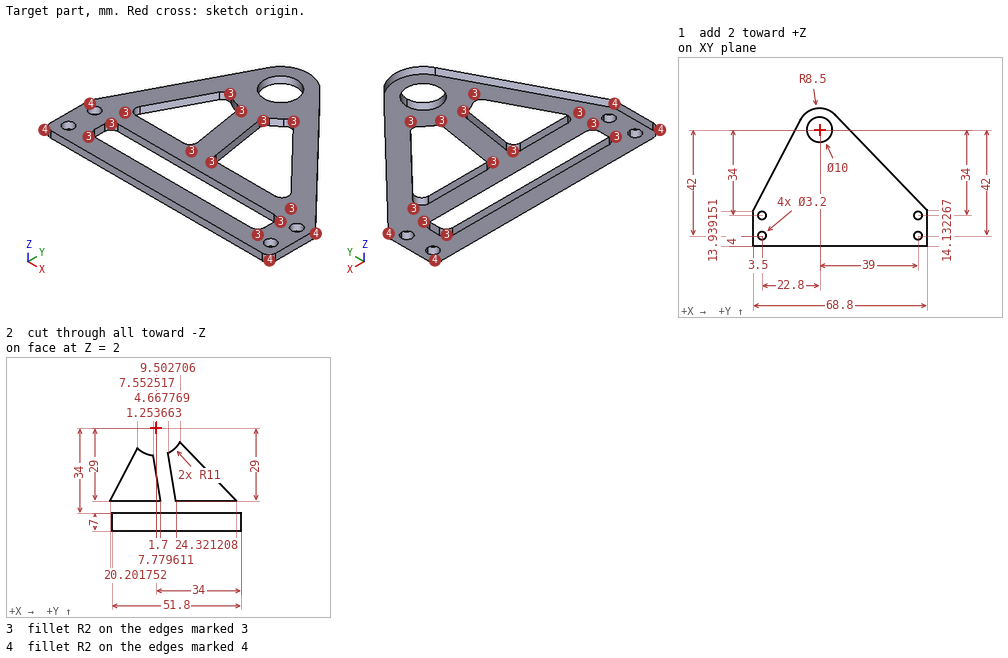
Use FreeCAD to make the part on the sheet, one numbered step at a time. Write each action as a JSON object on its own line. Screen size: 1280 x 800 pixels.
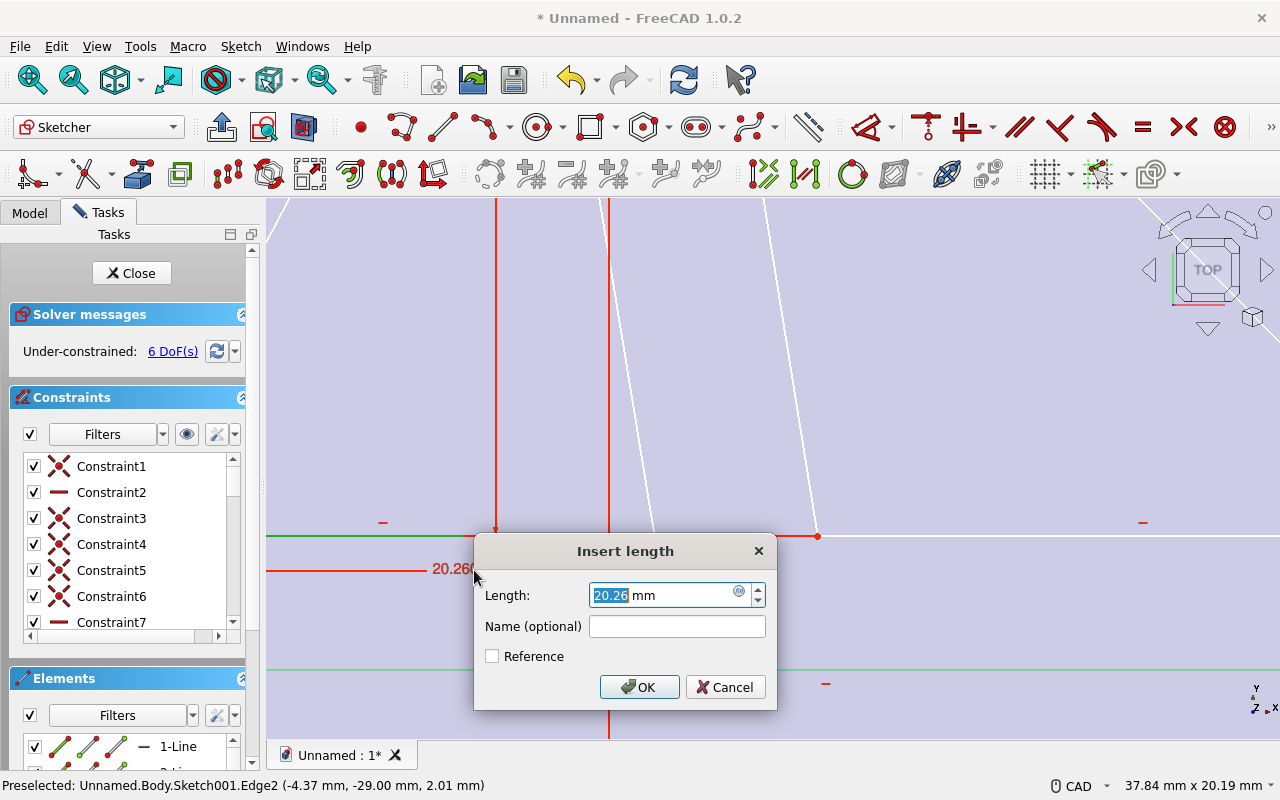
{"action": "type", "text": "20.201752"}
{"action": "key", "text": "Return"}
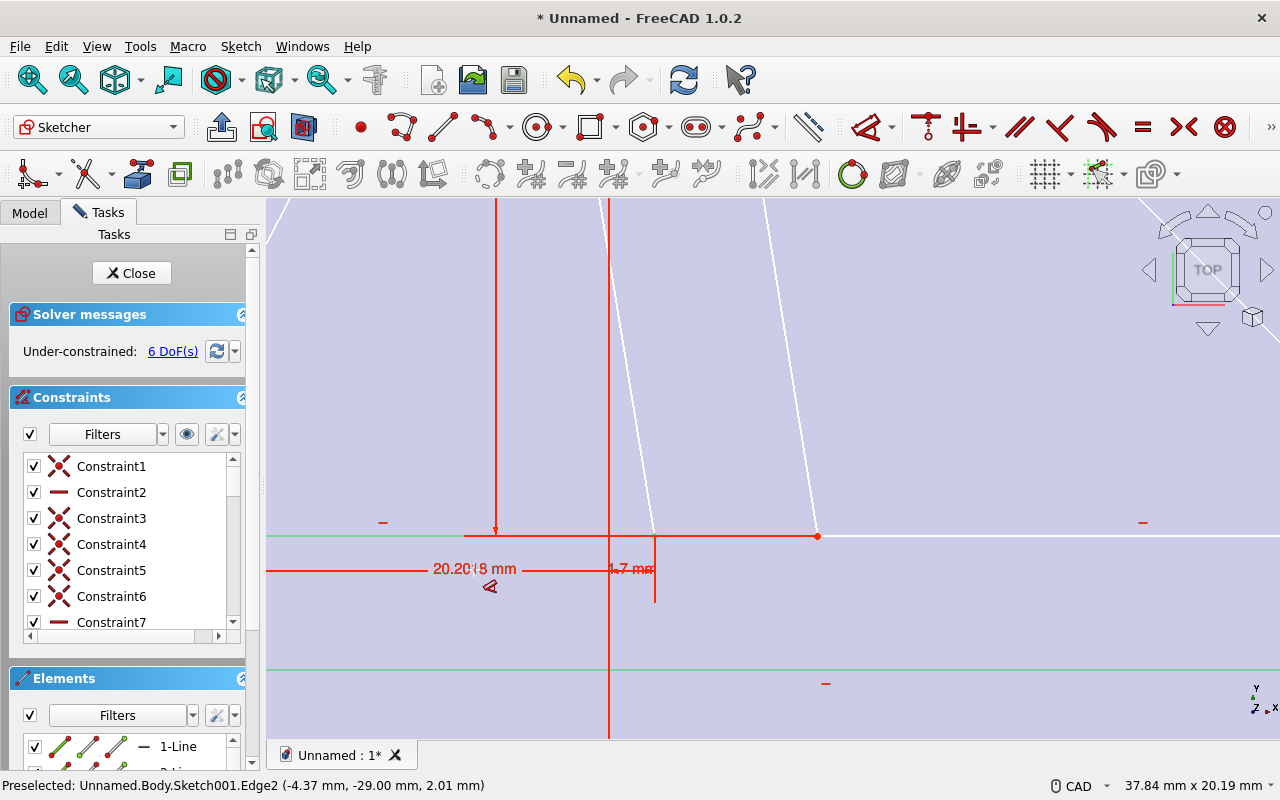
{"action": "left_click", "coordinate": [1013, 536]}
{"action": "left_click", "coordinate": [966, 570]}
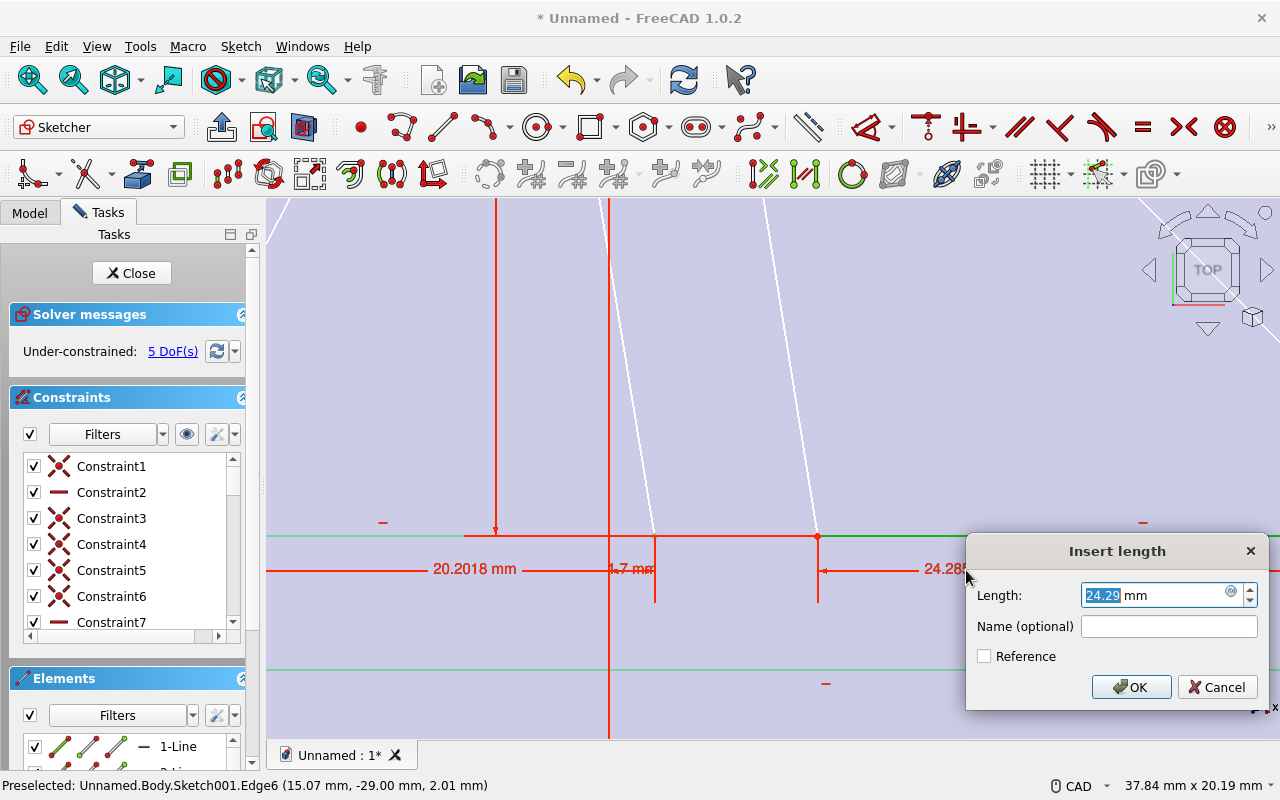
{"action": "type", "text": "24.321208"}
{"action": "key", "text": "Return"}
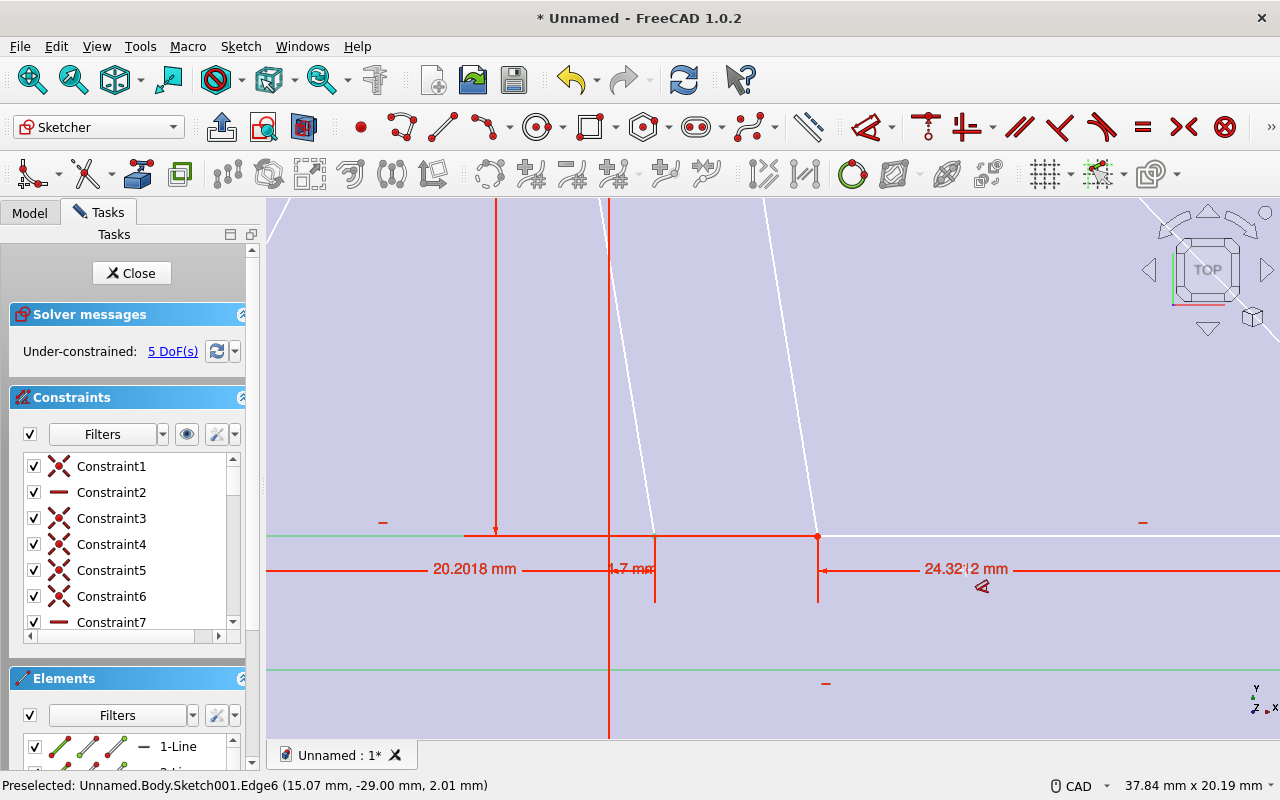
{"action": "scroll", "coordinate": [656, 537], "scroll_direction": "down", "scroll_amount": 6}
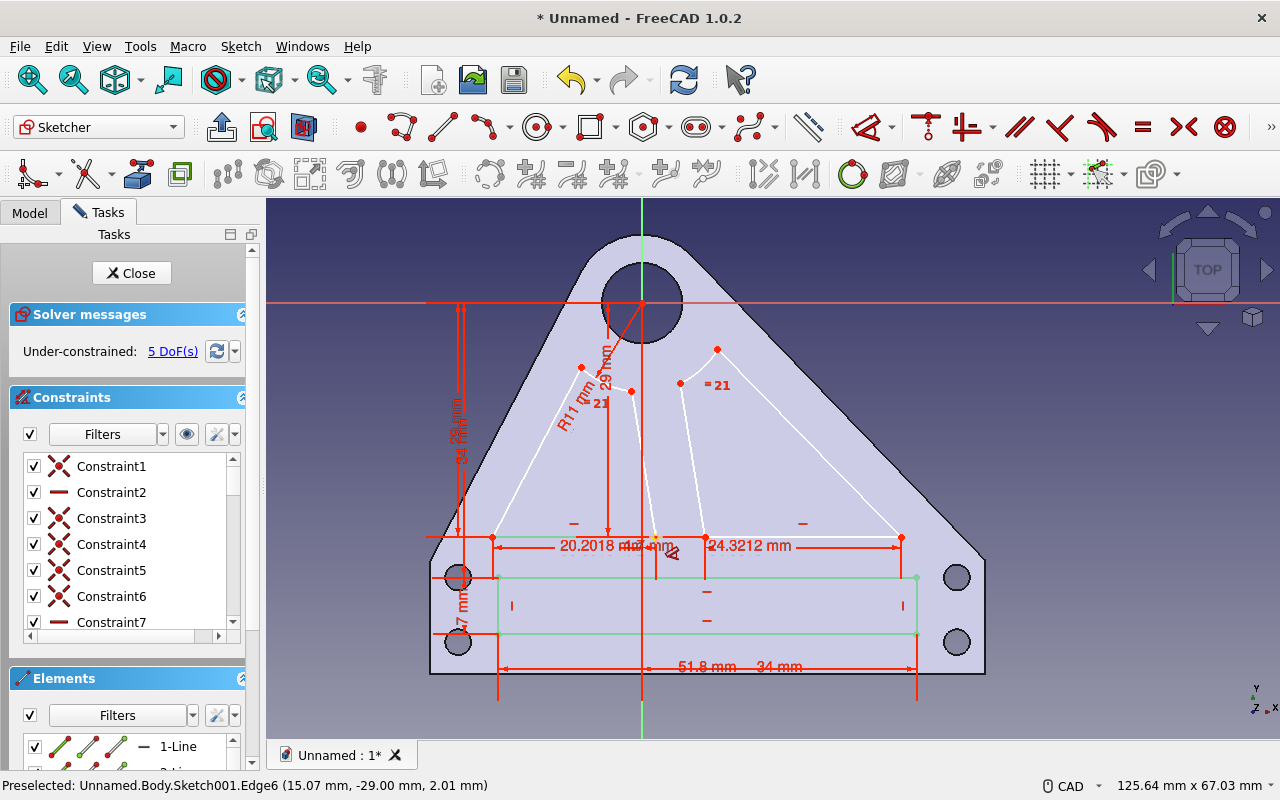
{"action": "left_click", "coordinate": [581, 368]}
{"action": "left_click", "coordinate": [612, 269]}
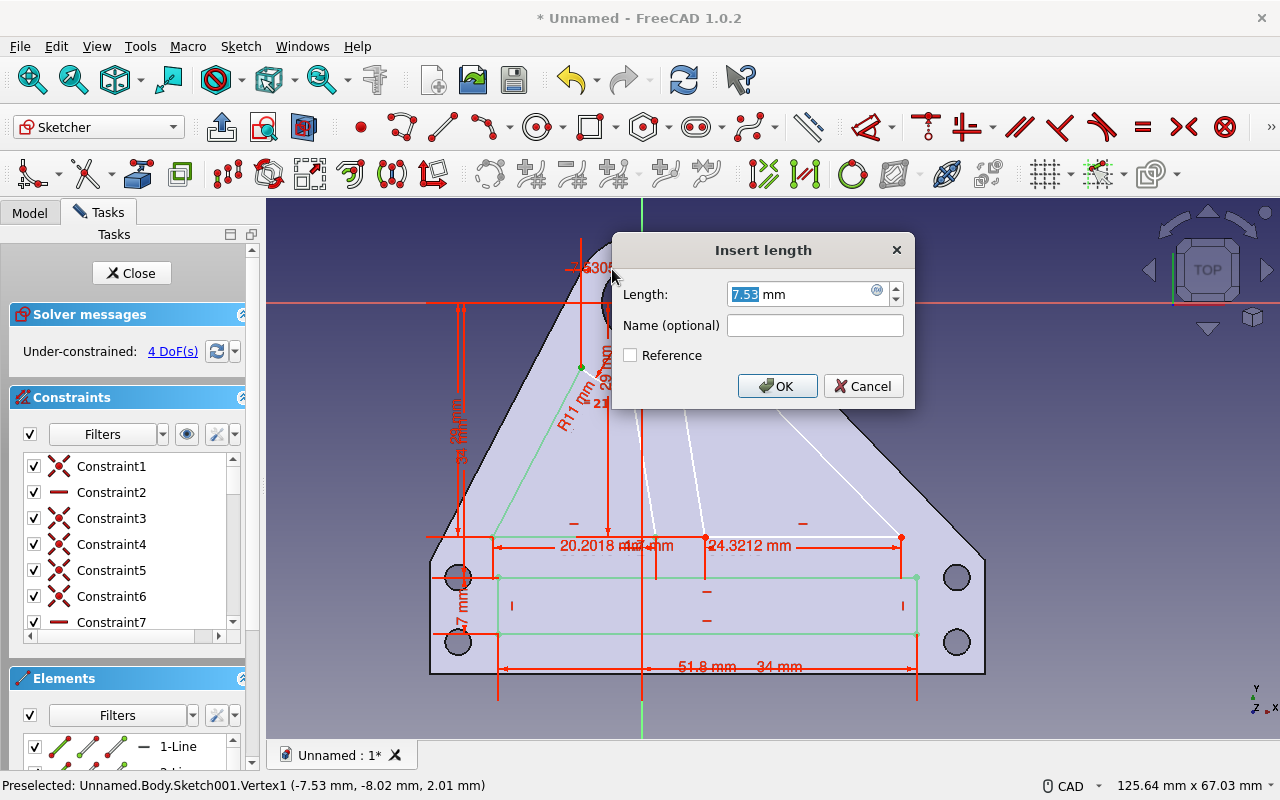
{"action": "type", "text": "7.552517"}
{"action": "key", "text": "Return"}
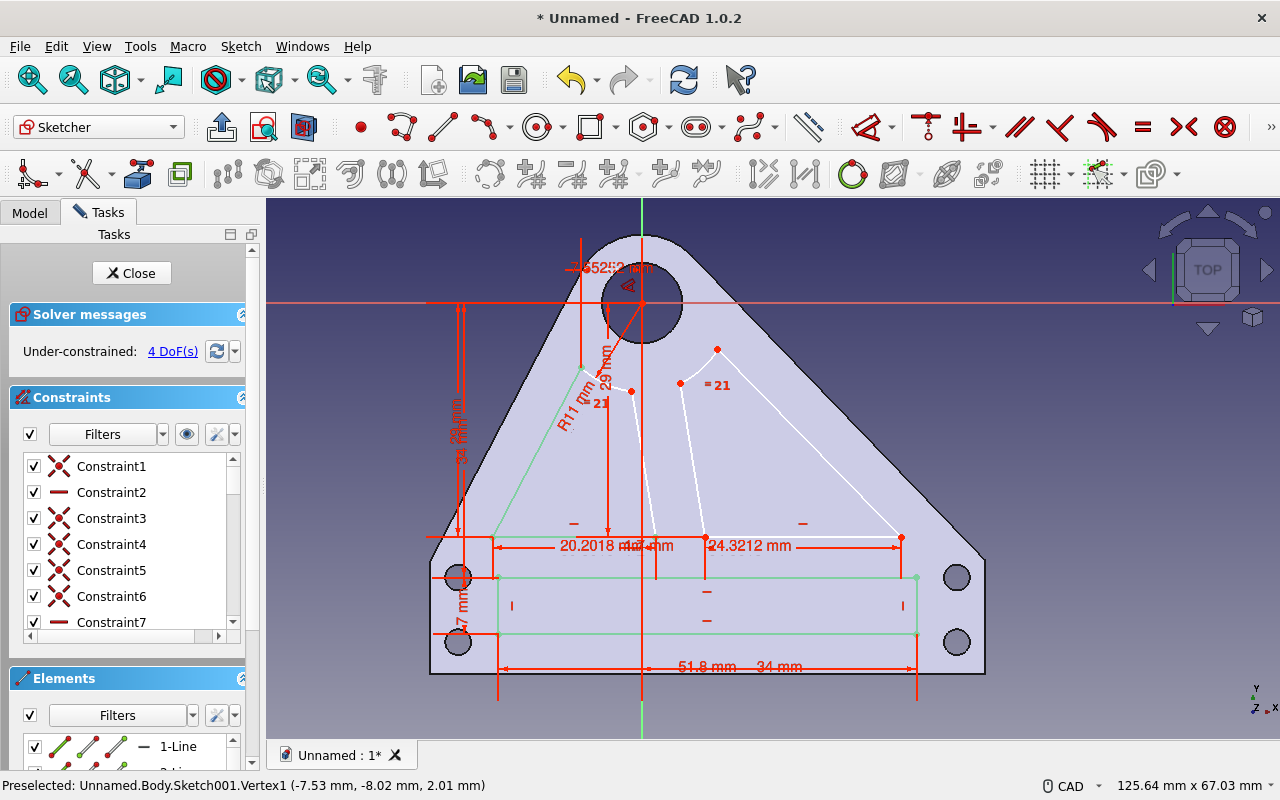
{"action": "scroll", "coordinate": [632, 391], "scroll_direction": "up", "scroll_amount": 7}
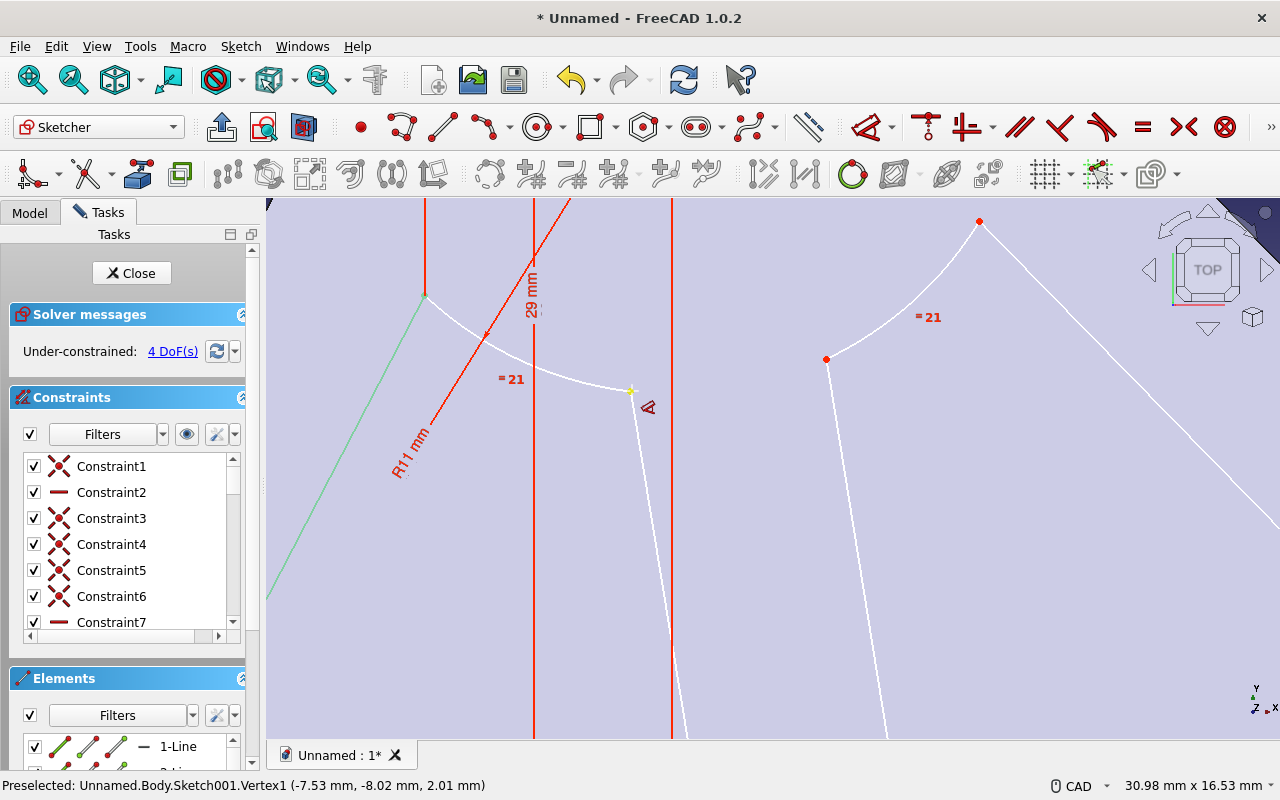
{"action": "left_click", "coordinate": [631, 391]}
{"action": "left_click", "coordinate": [651, 425]}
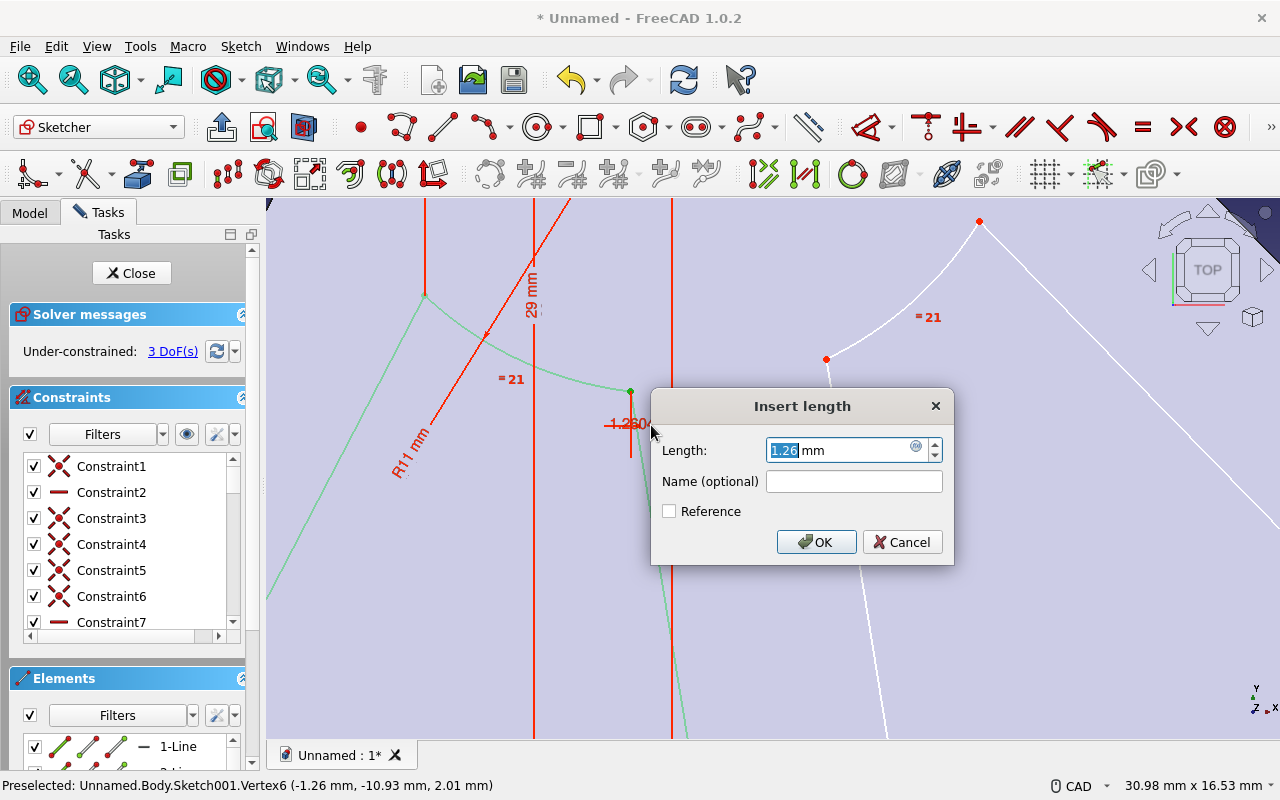
{"action": "type", "text": "1.253663"}
{"action": "key", "text": "Return"}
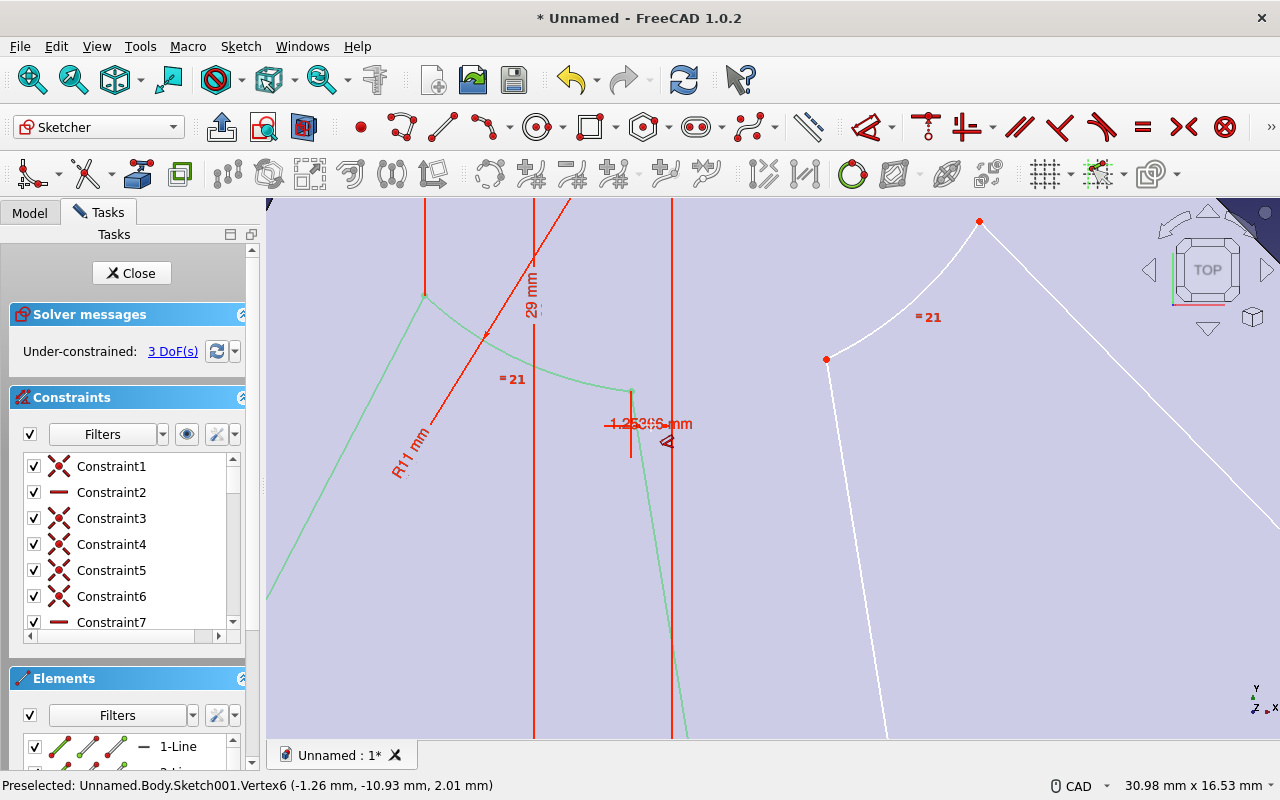
{"action": "scroll", "coordinate": [632, 391], "scroll_direction": "down", "scroll_amount": 7}